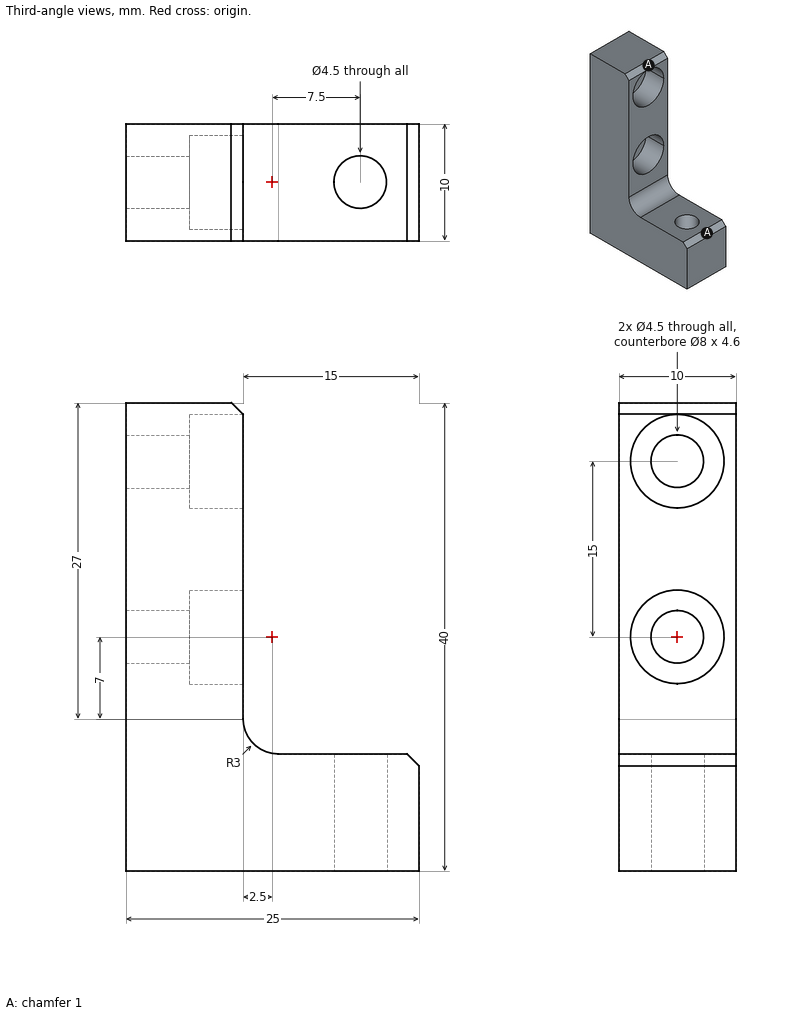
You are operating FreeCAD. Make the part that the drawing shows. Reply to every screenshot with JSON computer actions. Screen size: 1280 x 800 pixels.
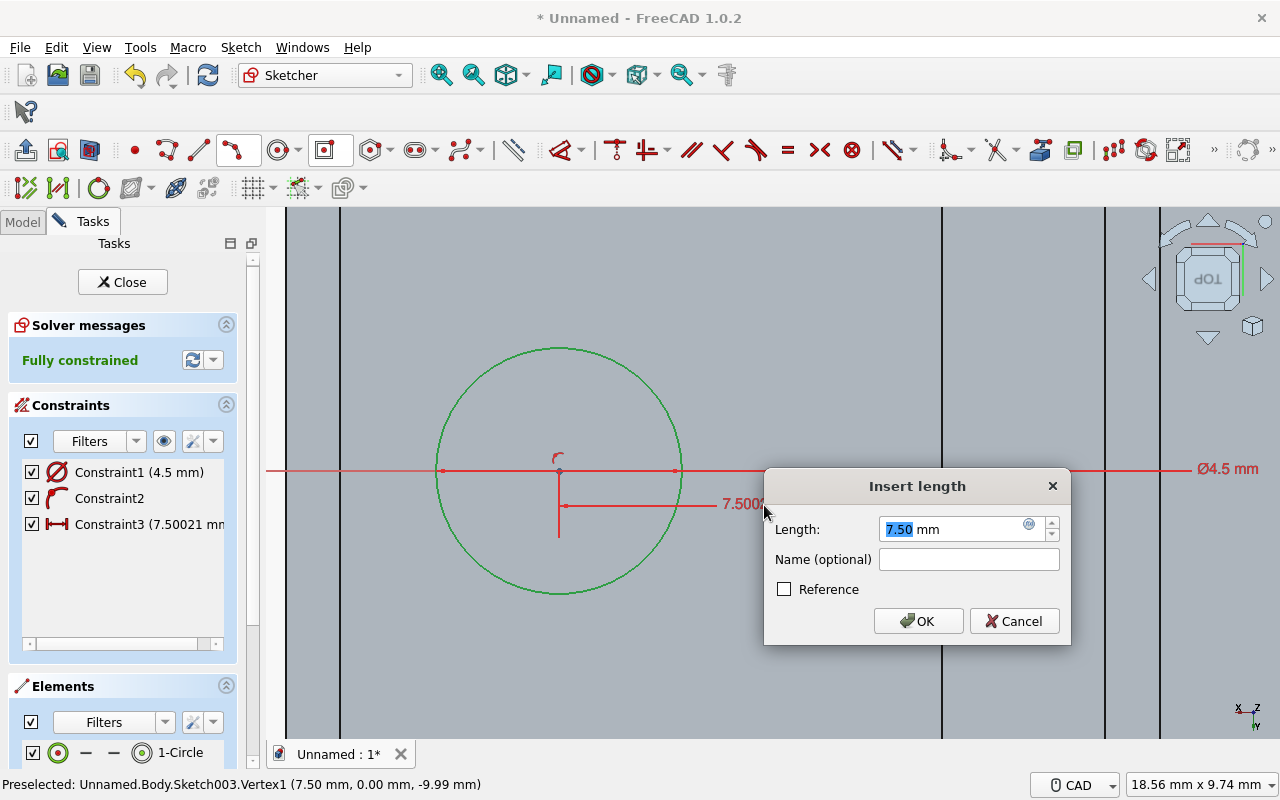
{"action": "type", "text": "7.5"}
{"action": "key", "text": "Return"}
{"action": "key", "text": "Escape"}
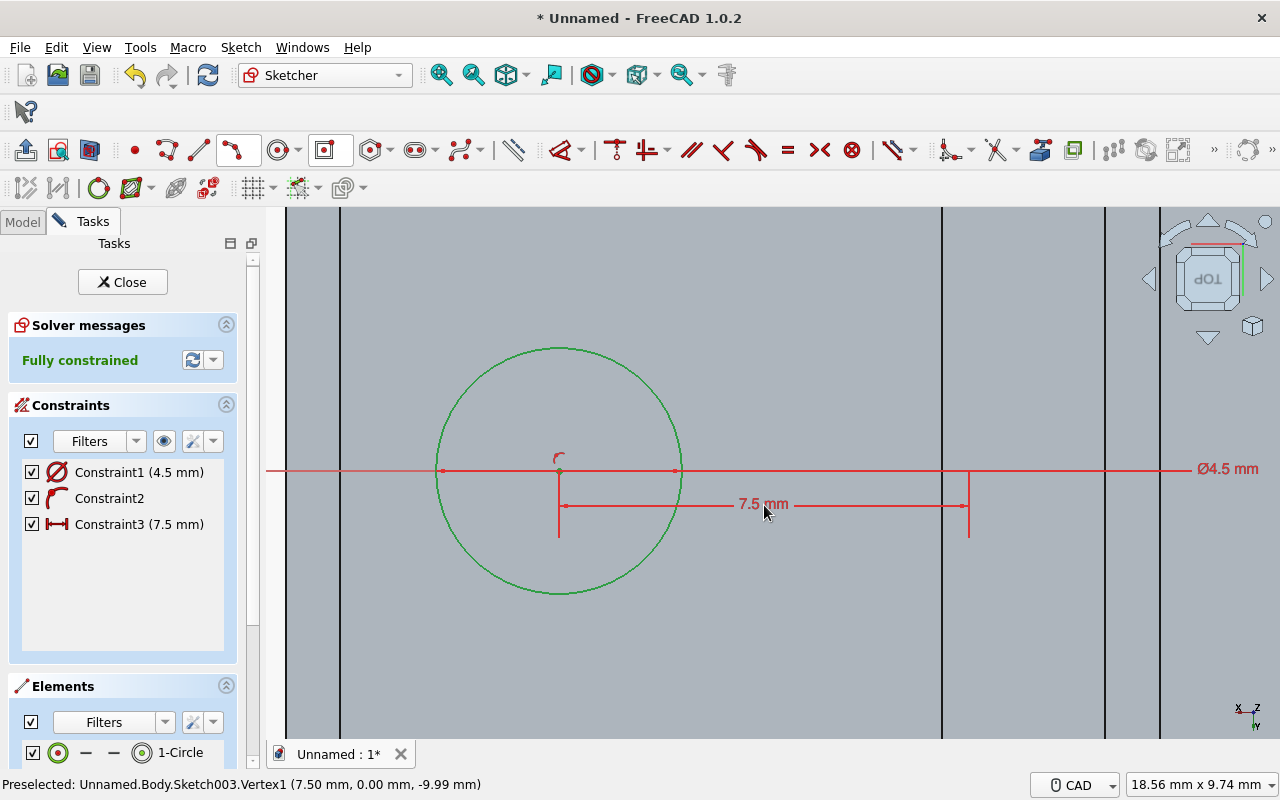
{"action": "left_click", "coordinate": [123, 282]}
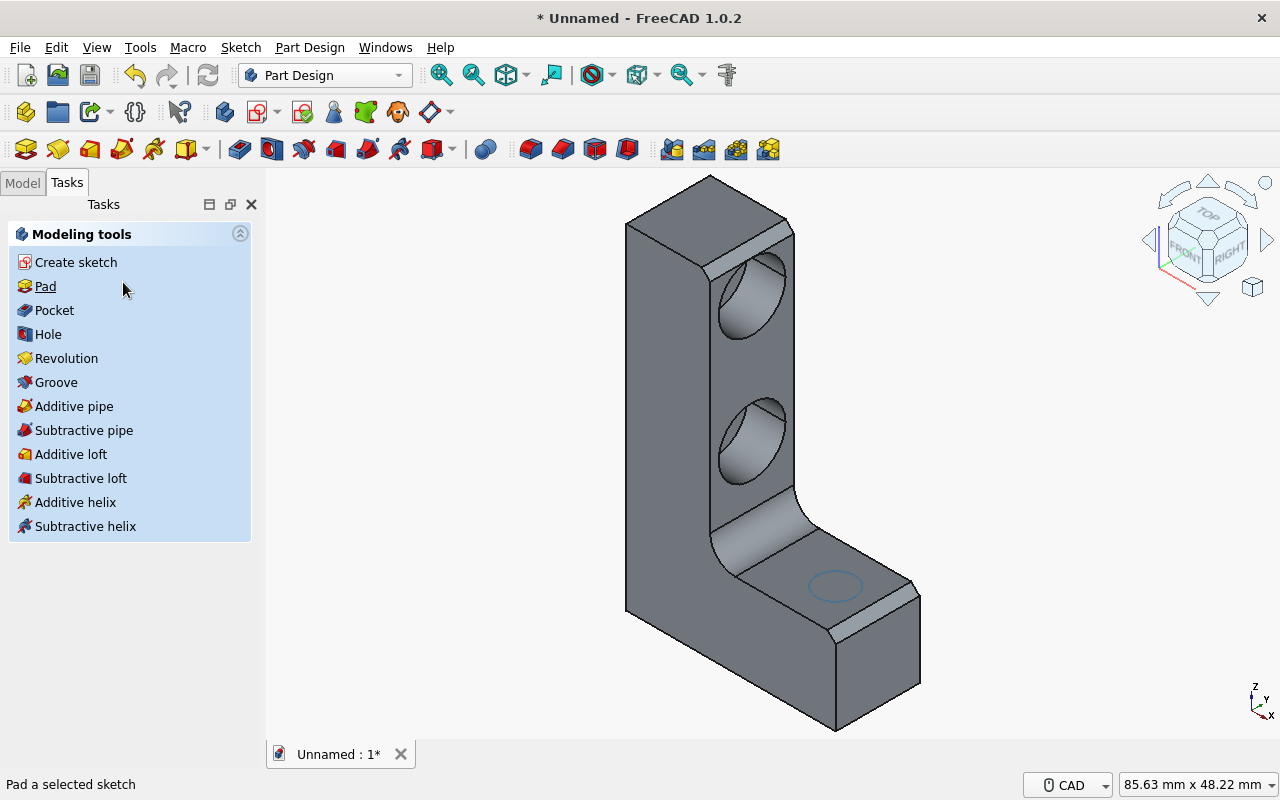
{"action": "left_click", "coordinate": [272, 150]}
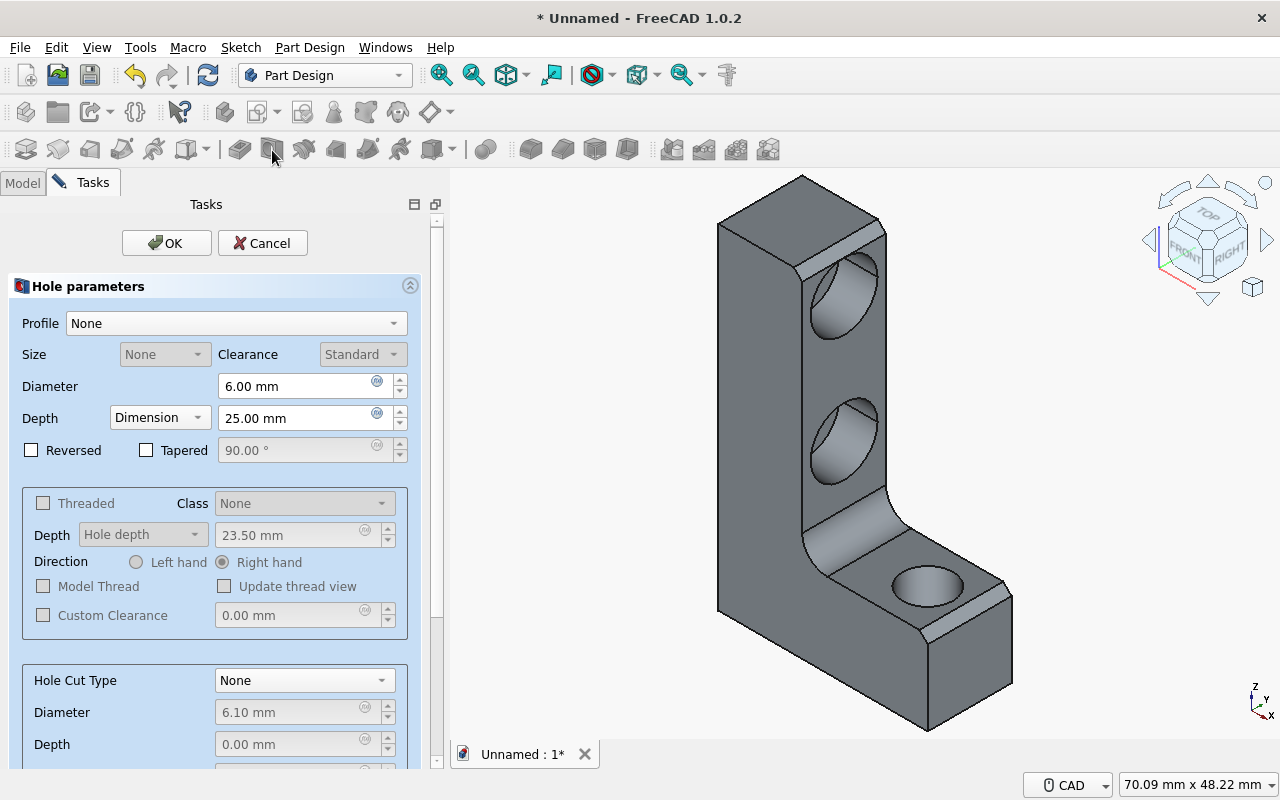
{"action": "triple_click", "coordinate": [305, 386]}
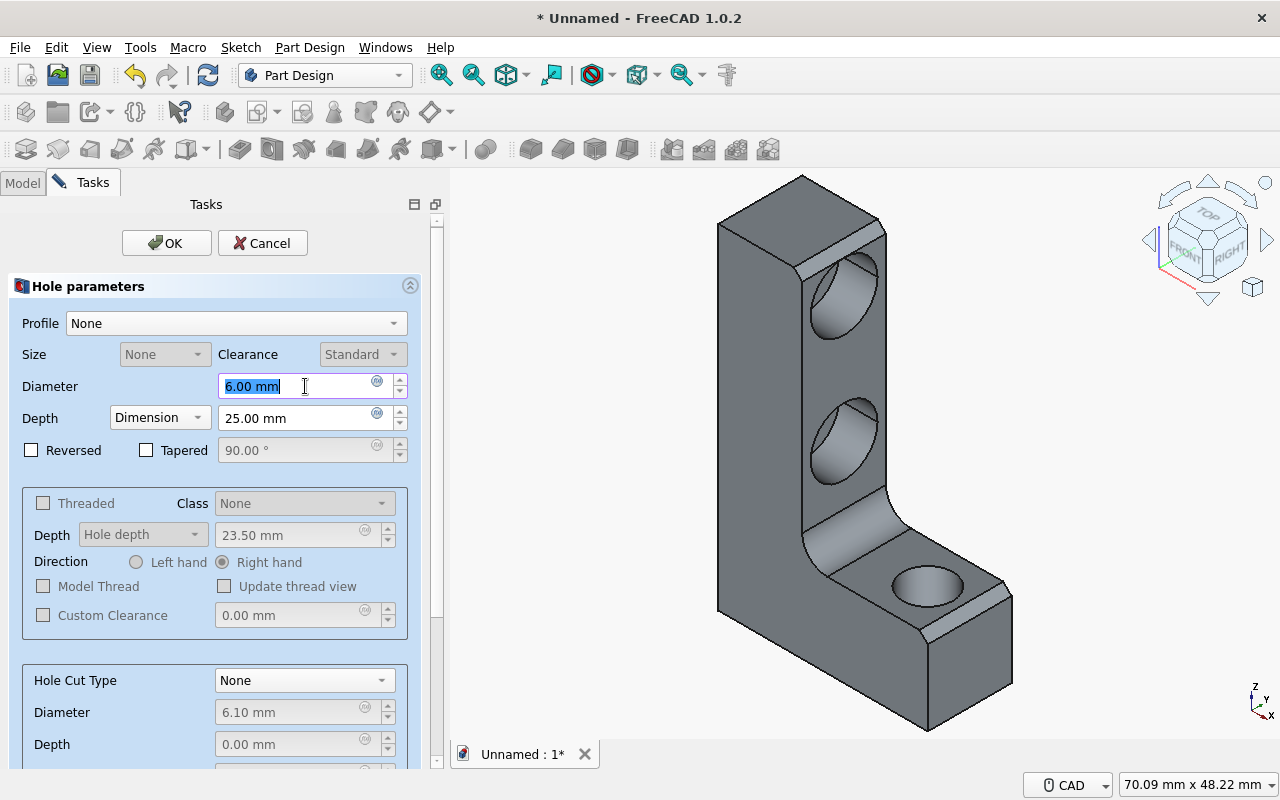
{"action": "type", "text": "4.5"}
{"action": "key", "text": "Tab"}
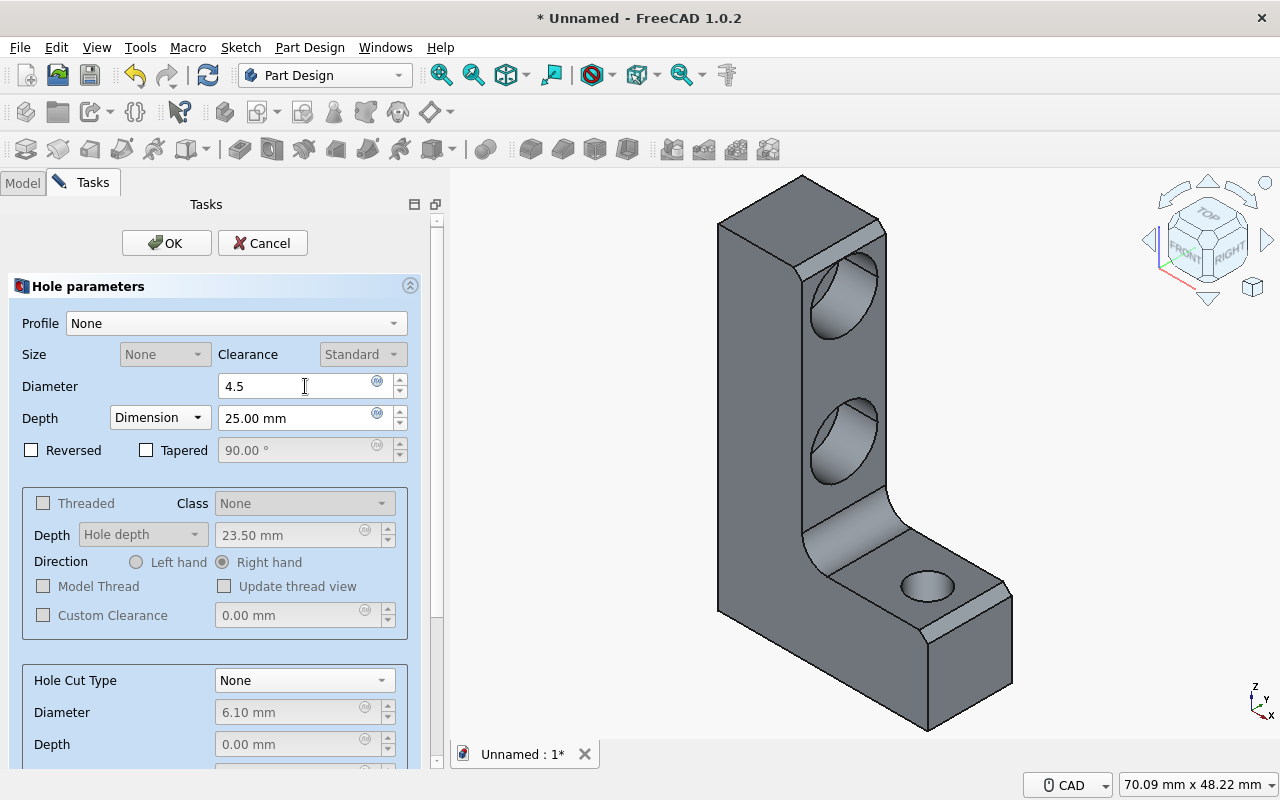
{"action": "left_click", "coordinate": [161, 418]}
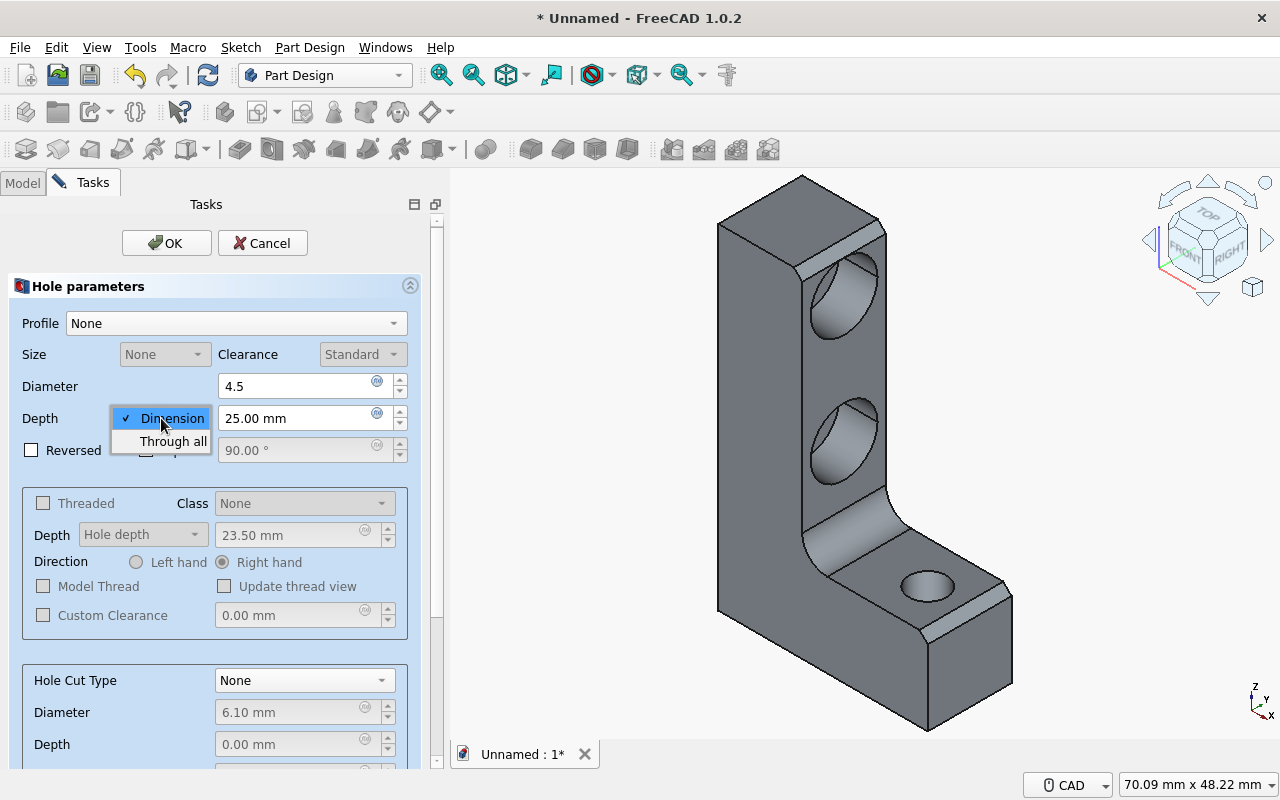
{"action": "left_click", "coordinate": [160, 442]}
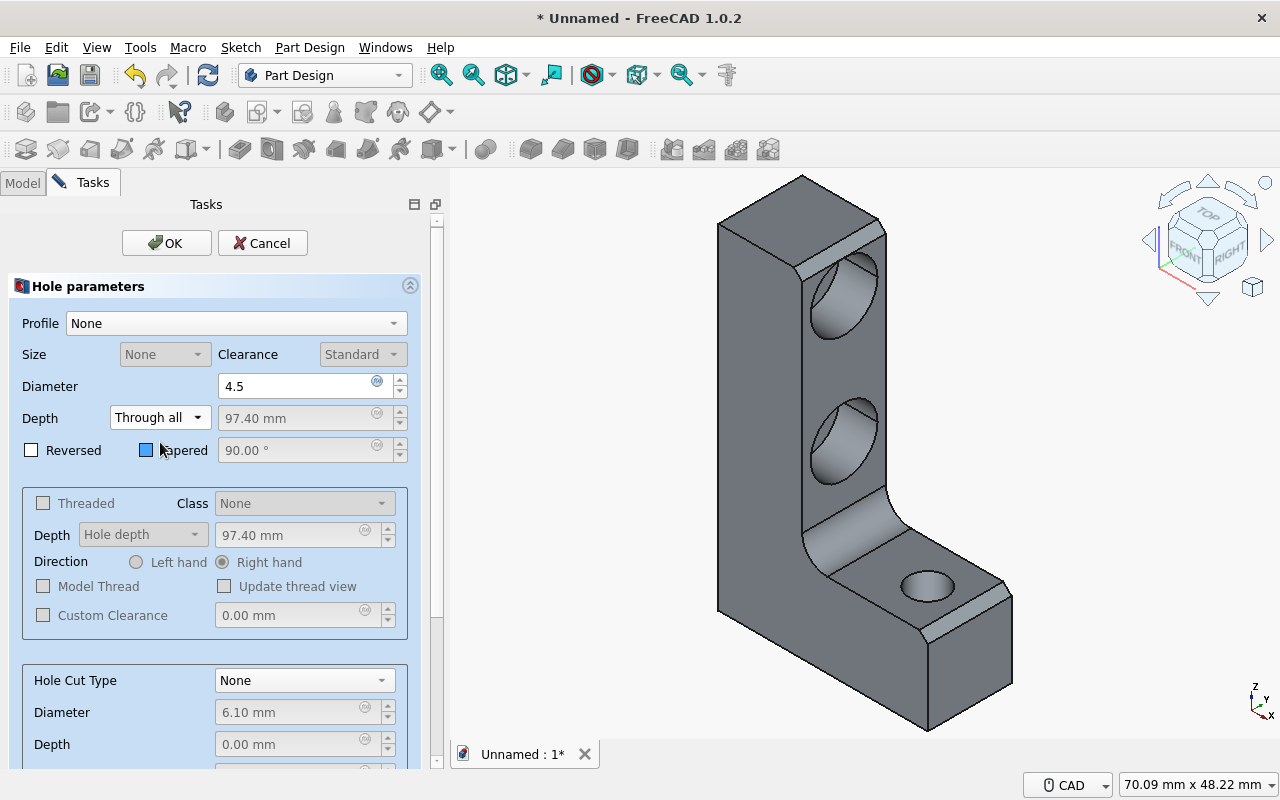
{"action": "left_click", "coordinate": [167, 243]}